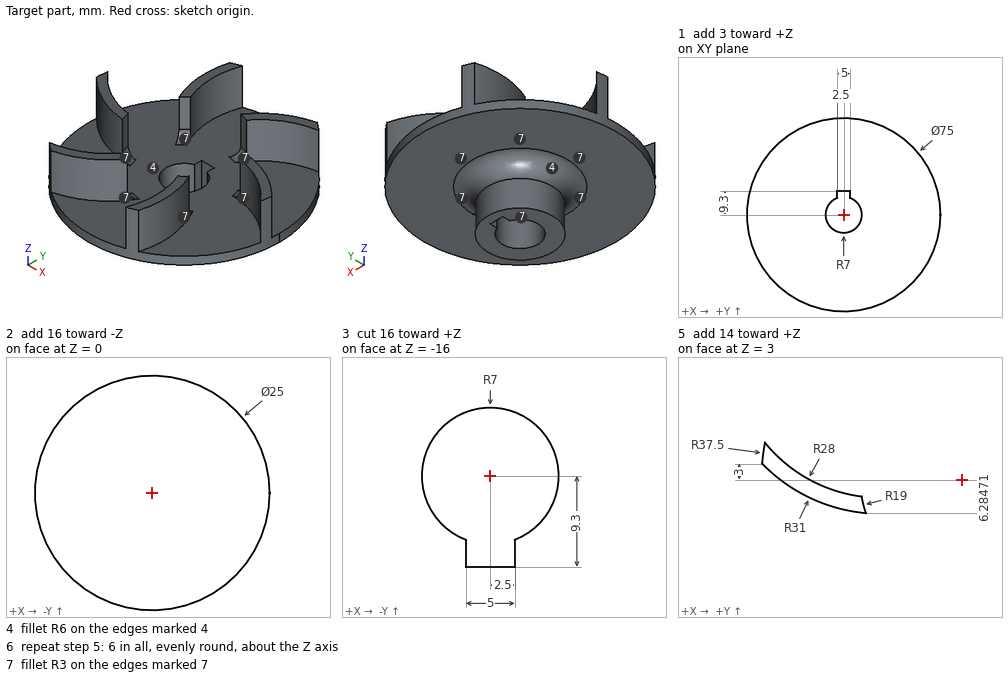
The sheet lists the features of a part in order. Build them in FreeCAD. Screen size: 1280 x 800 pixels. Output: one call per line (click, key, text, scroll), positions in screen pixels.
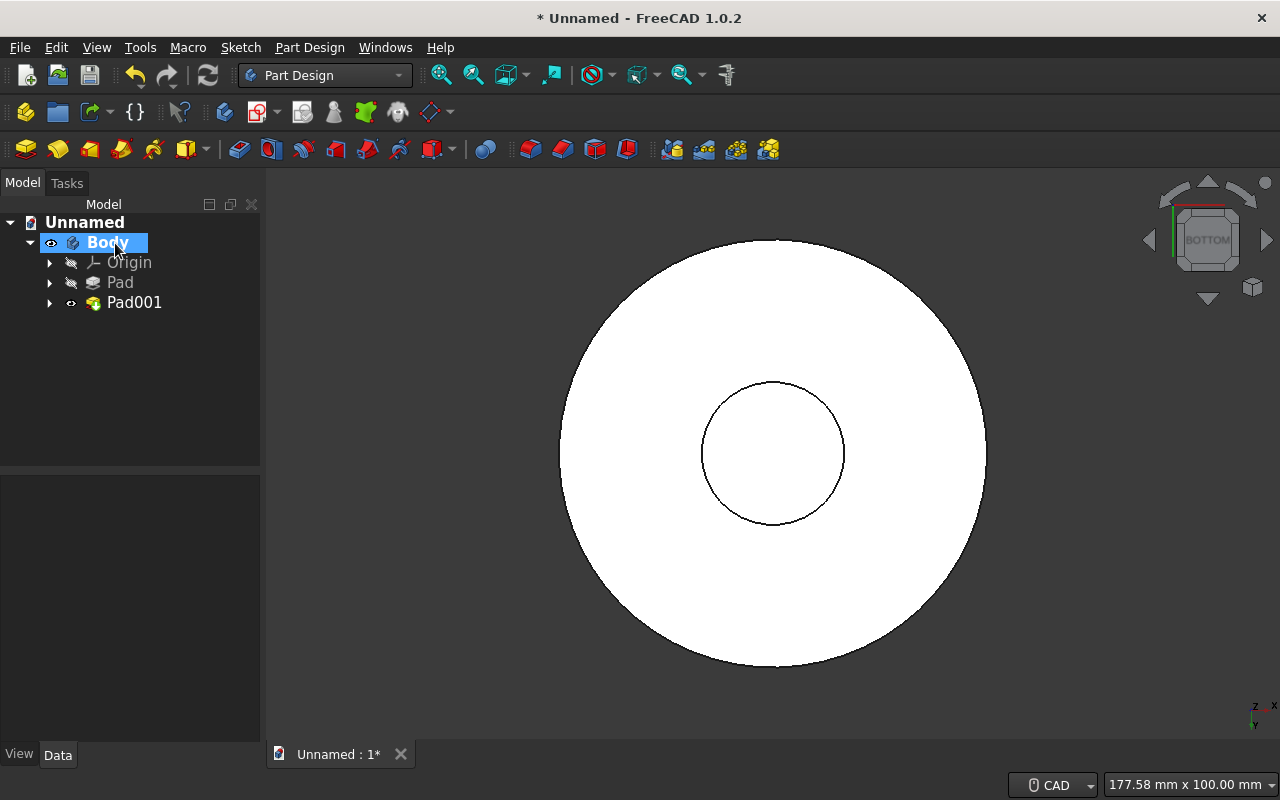
click(773, 453)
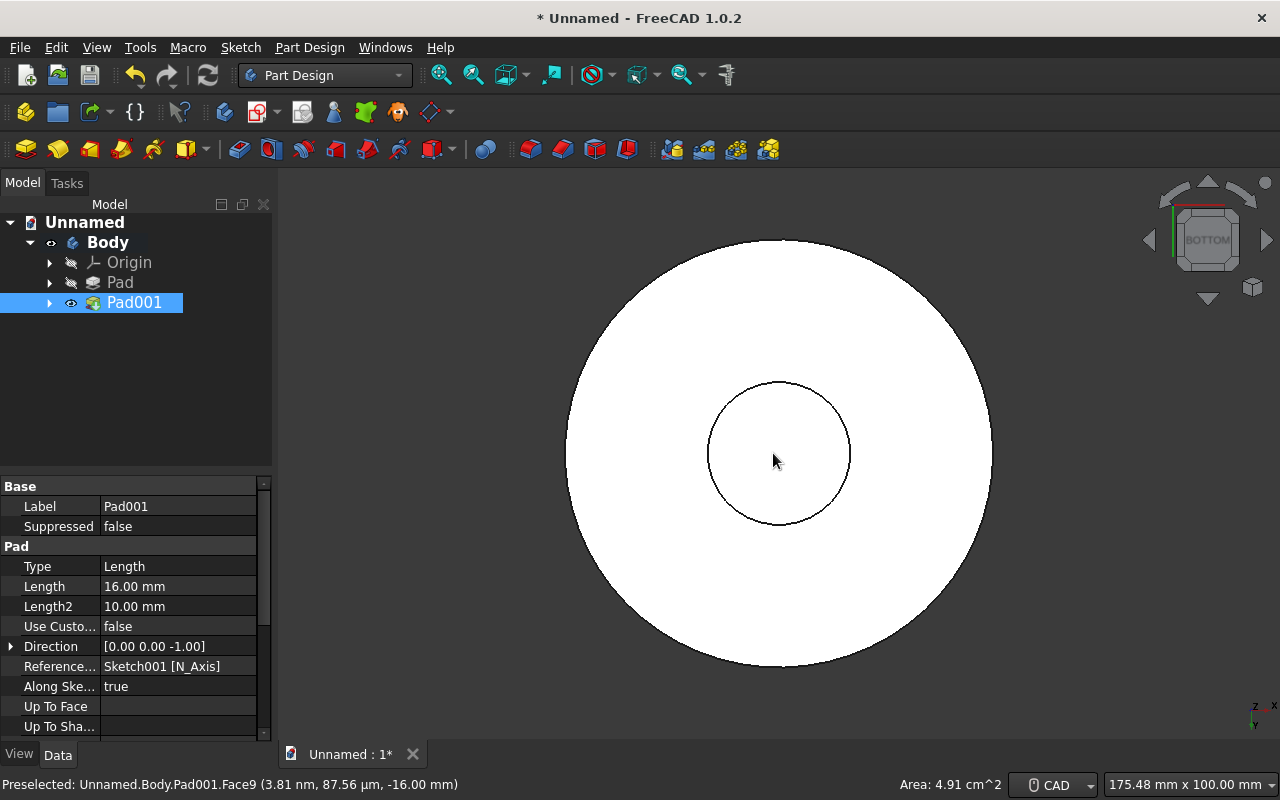
click(258, 112)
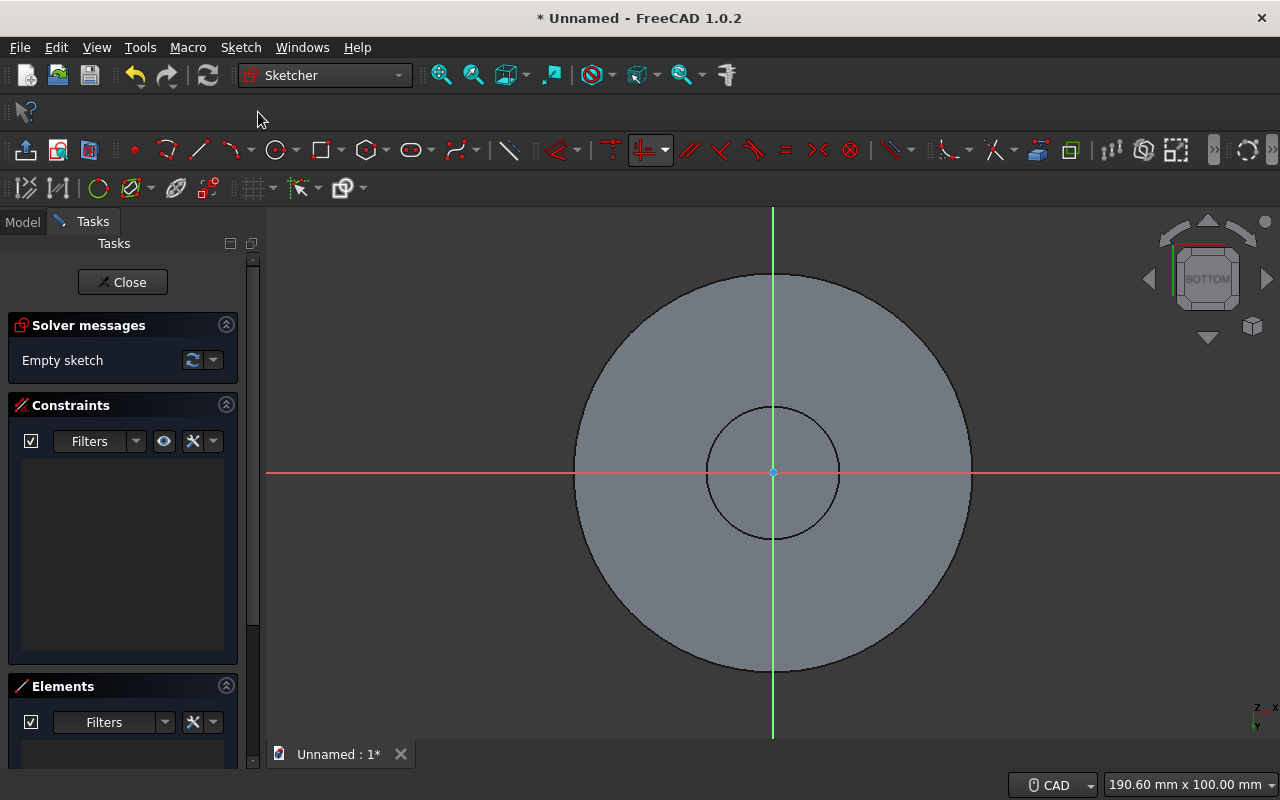
scroll(795, 481, up, 7)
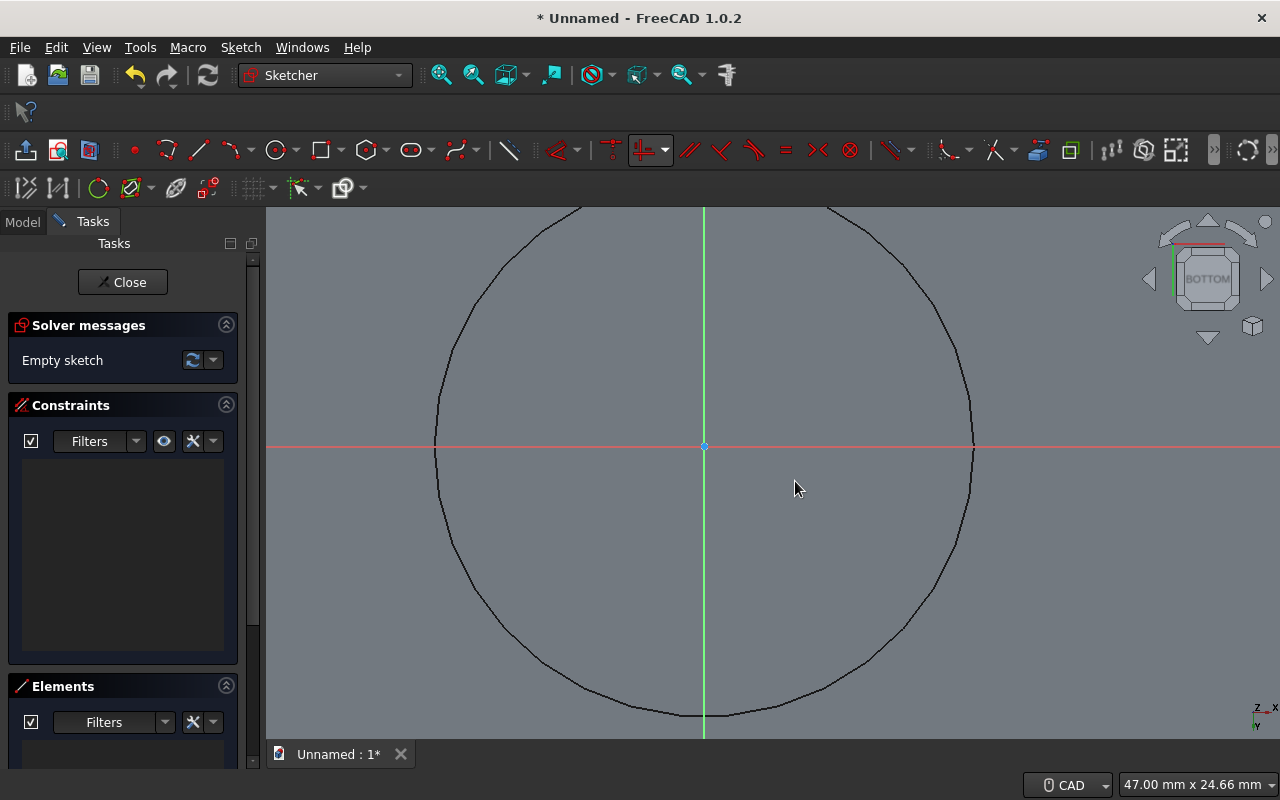
click(168, 150)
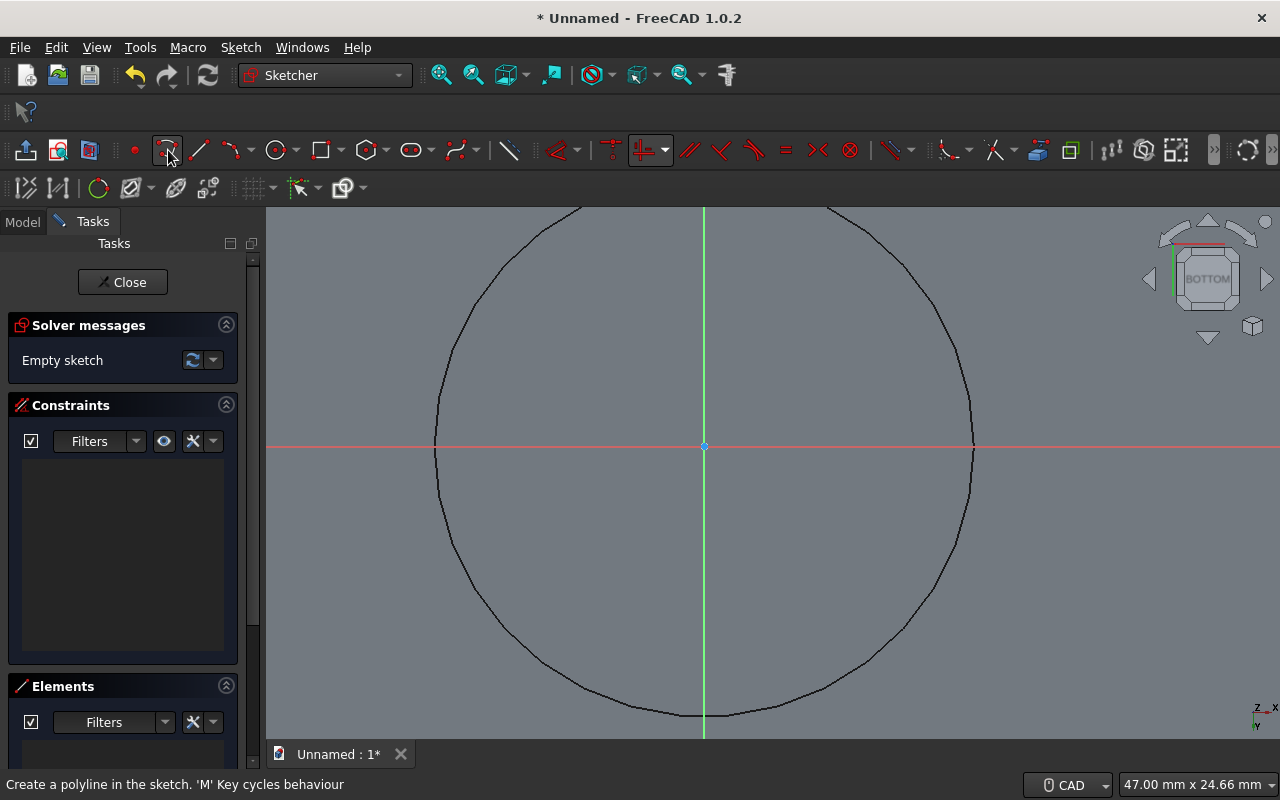
click(758, 588)
click(758, 648)
click(650, 648)
click(650, 588)
right_click(650, 588)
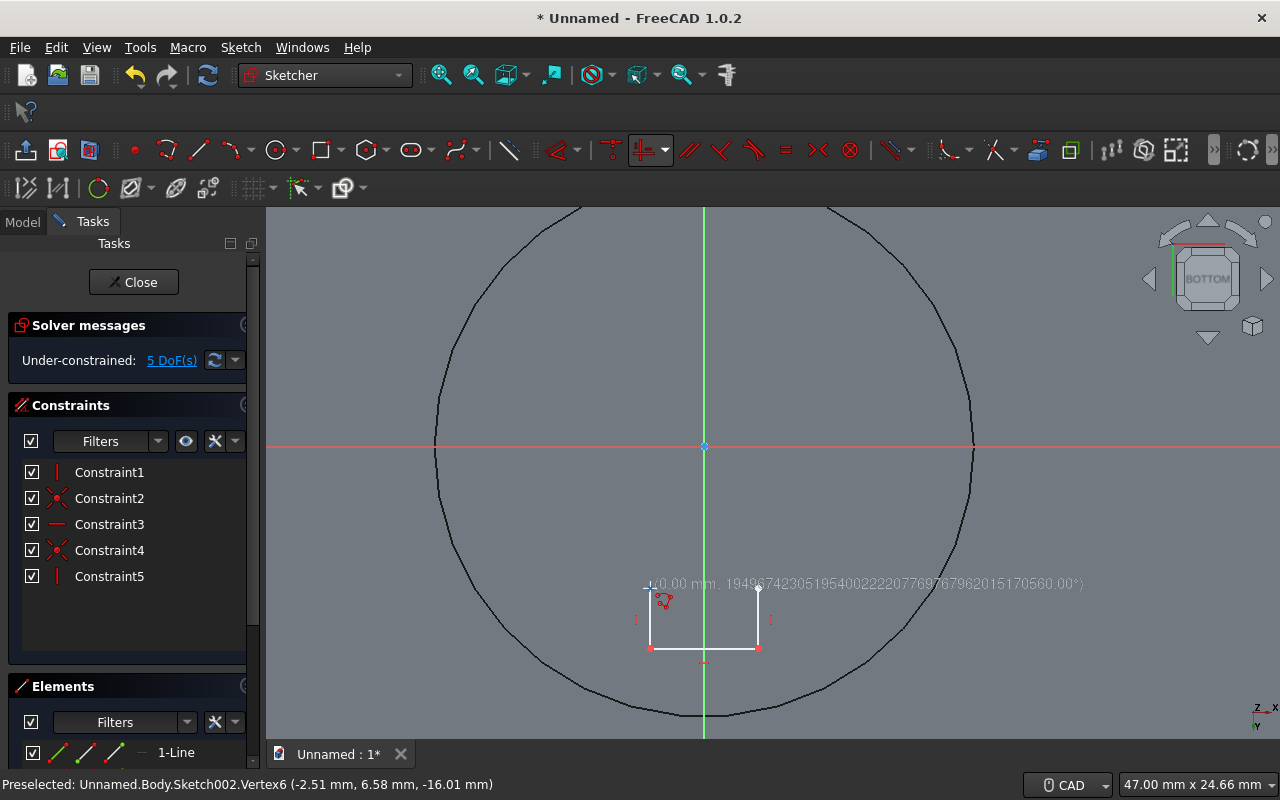
key(g)
key(3)
key(a)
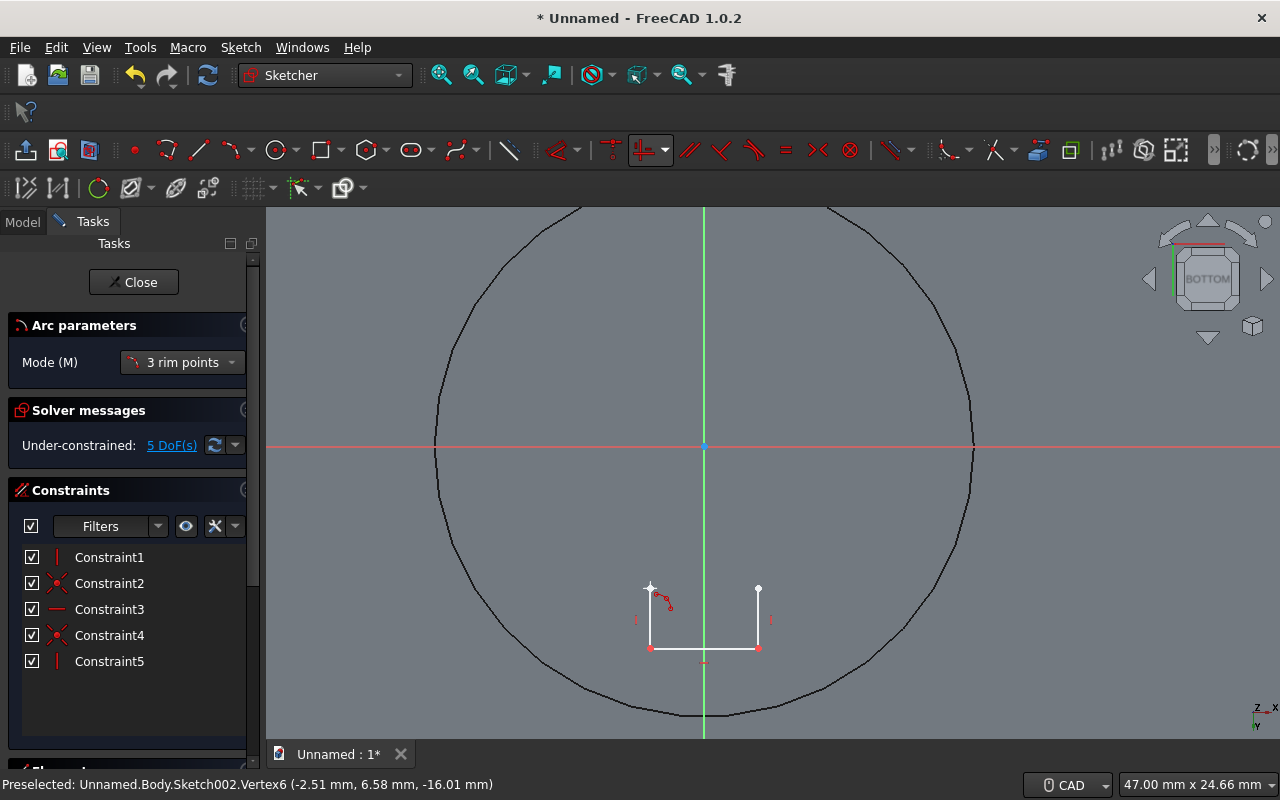
click(650, 589)
click(758, 589)
click(784, 319)
key(Escape)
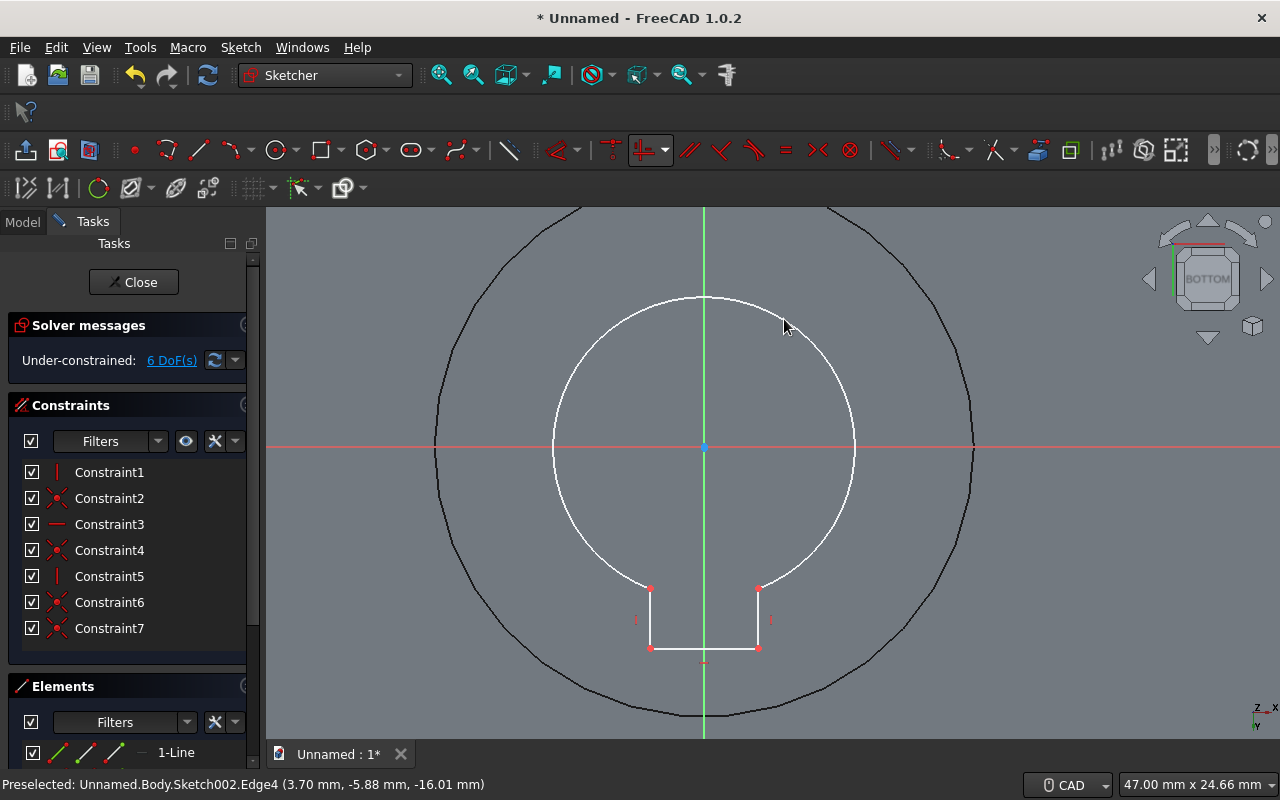
drag(694, 437, 714, 458)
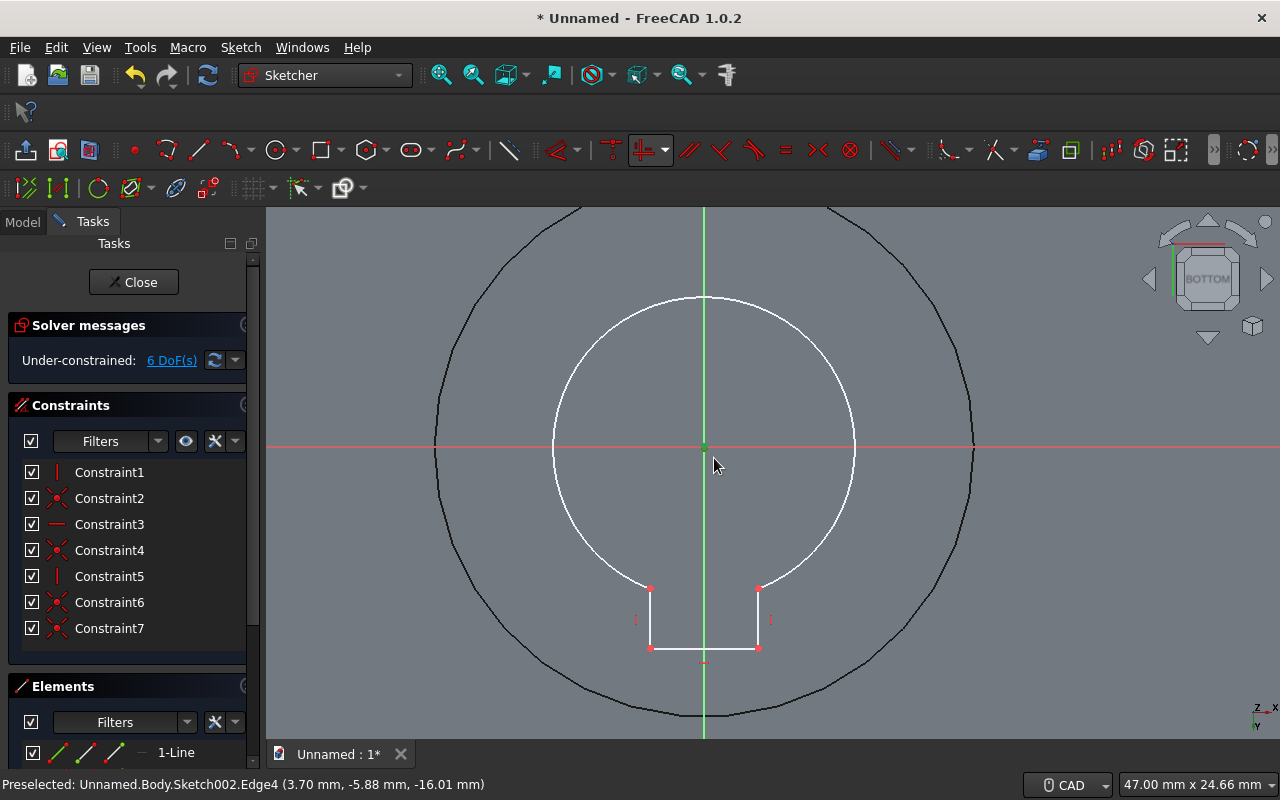
key(c)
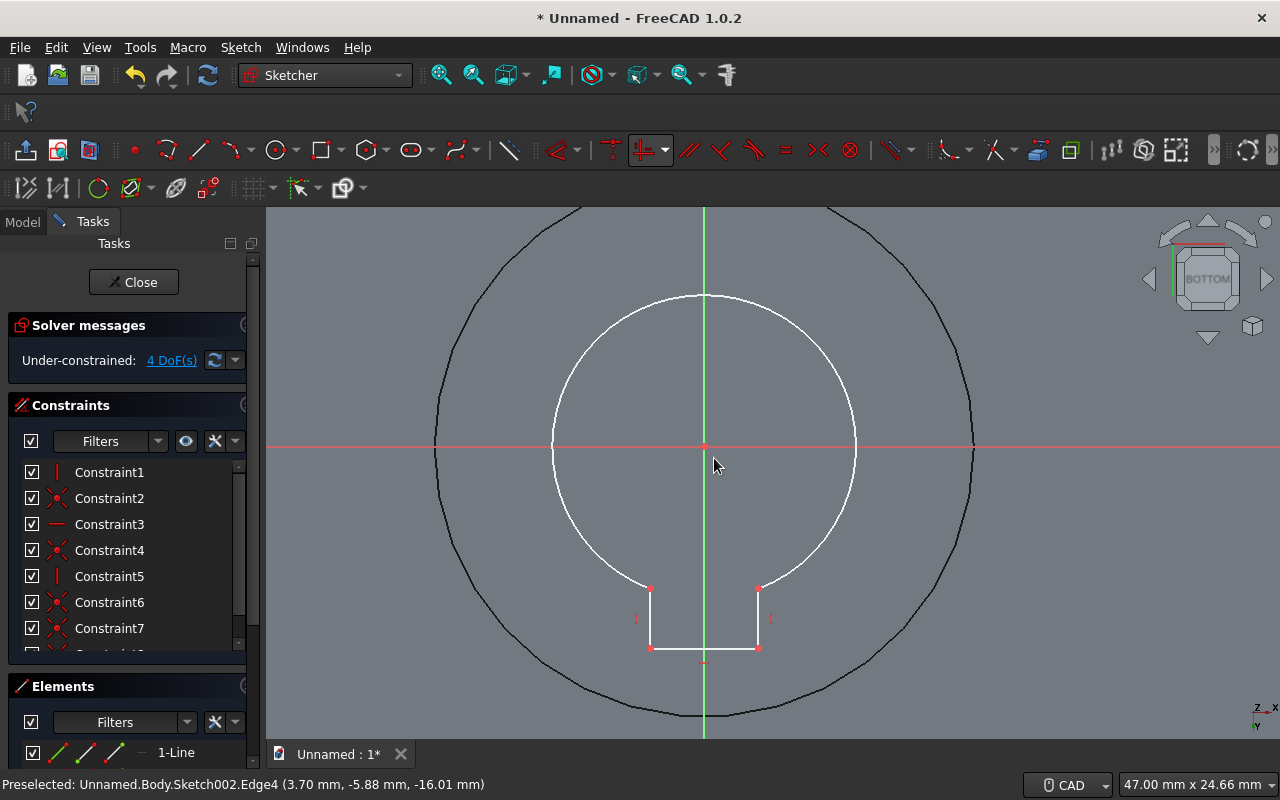
click(840, 380)